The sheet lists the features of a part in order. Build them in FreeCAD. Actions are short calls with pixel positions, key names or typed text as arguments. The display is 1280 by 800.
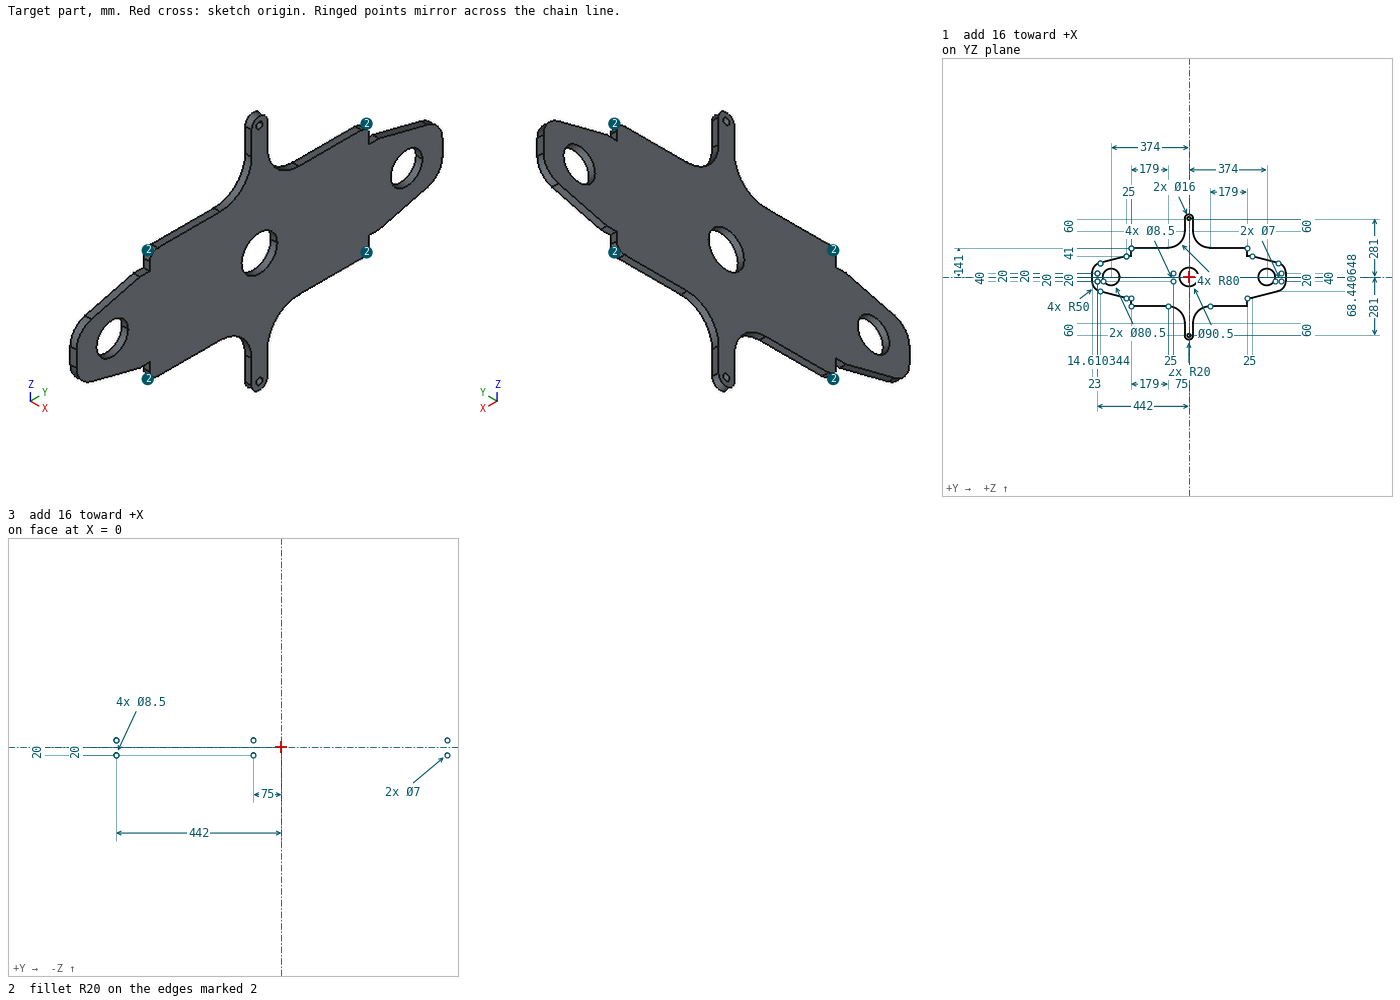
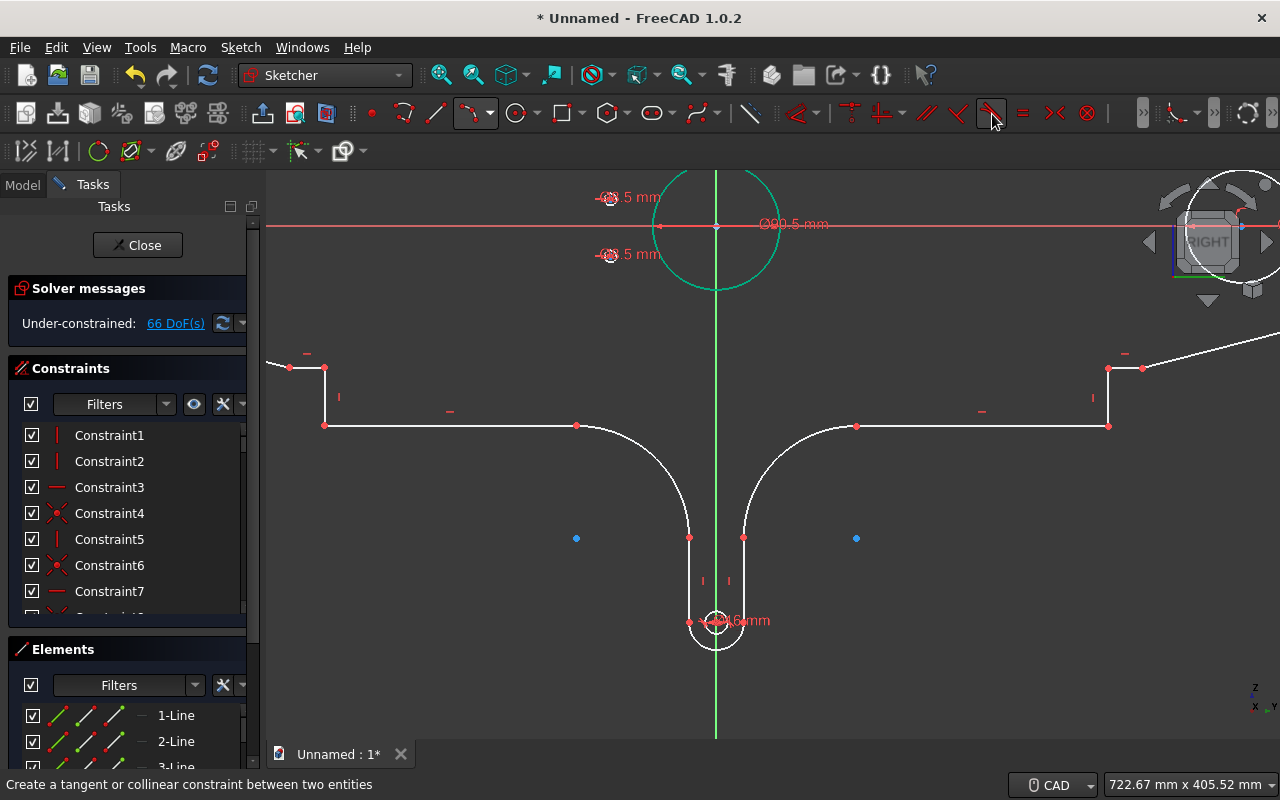
scroll(695, 641, down, 4)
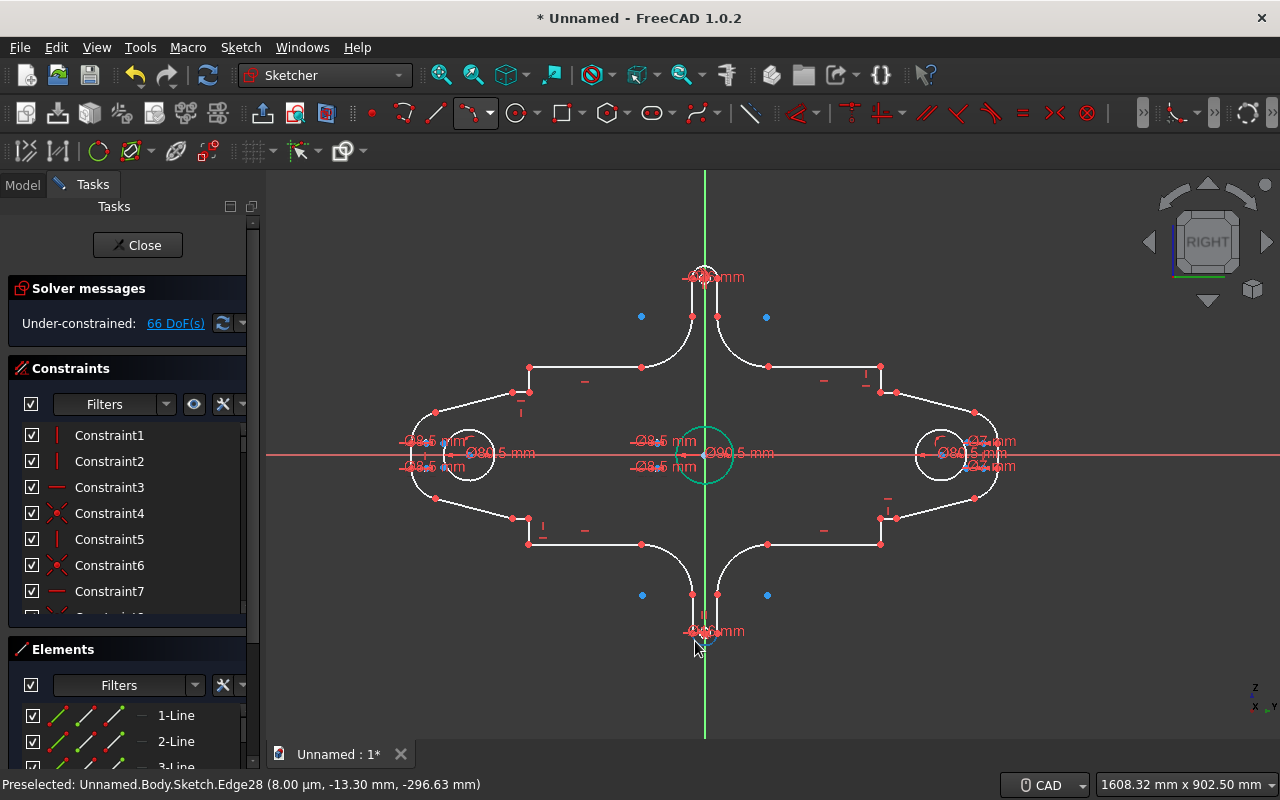
click(424, 418)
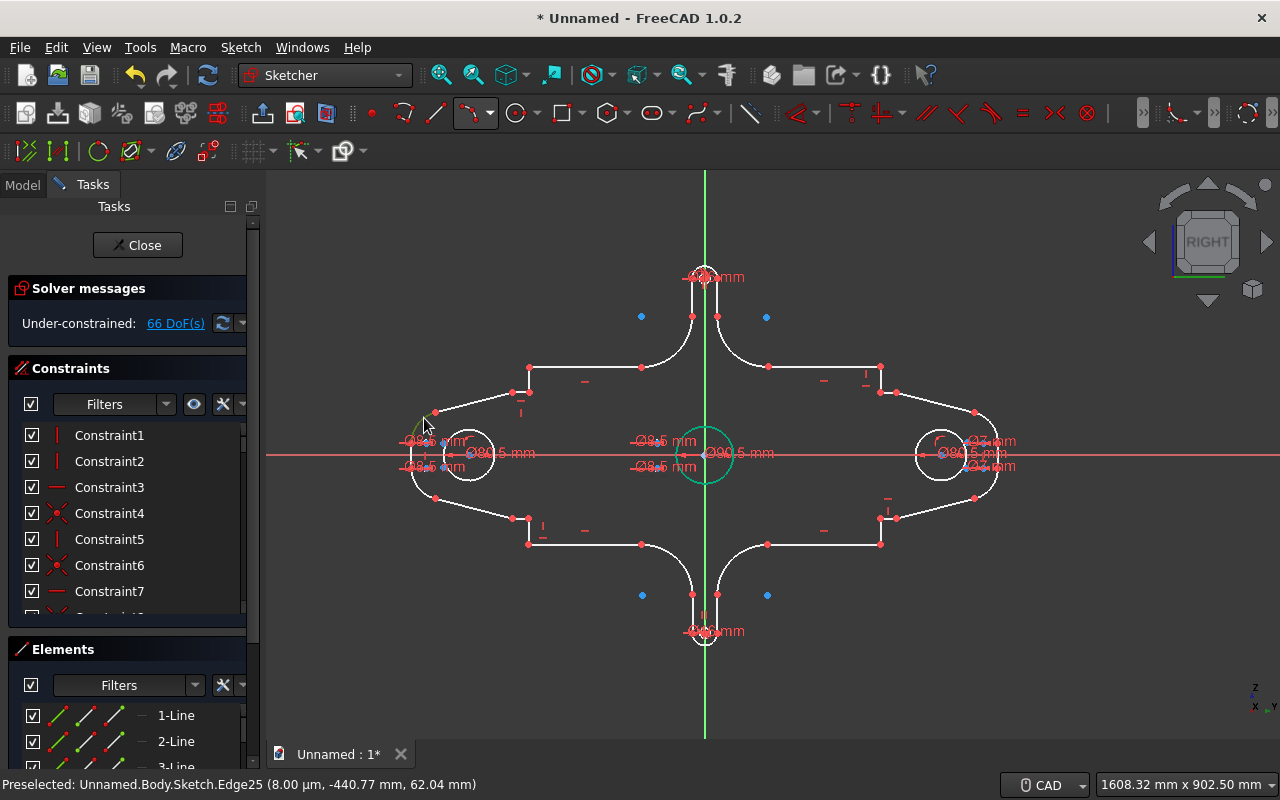
click(414, 481)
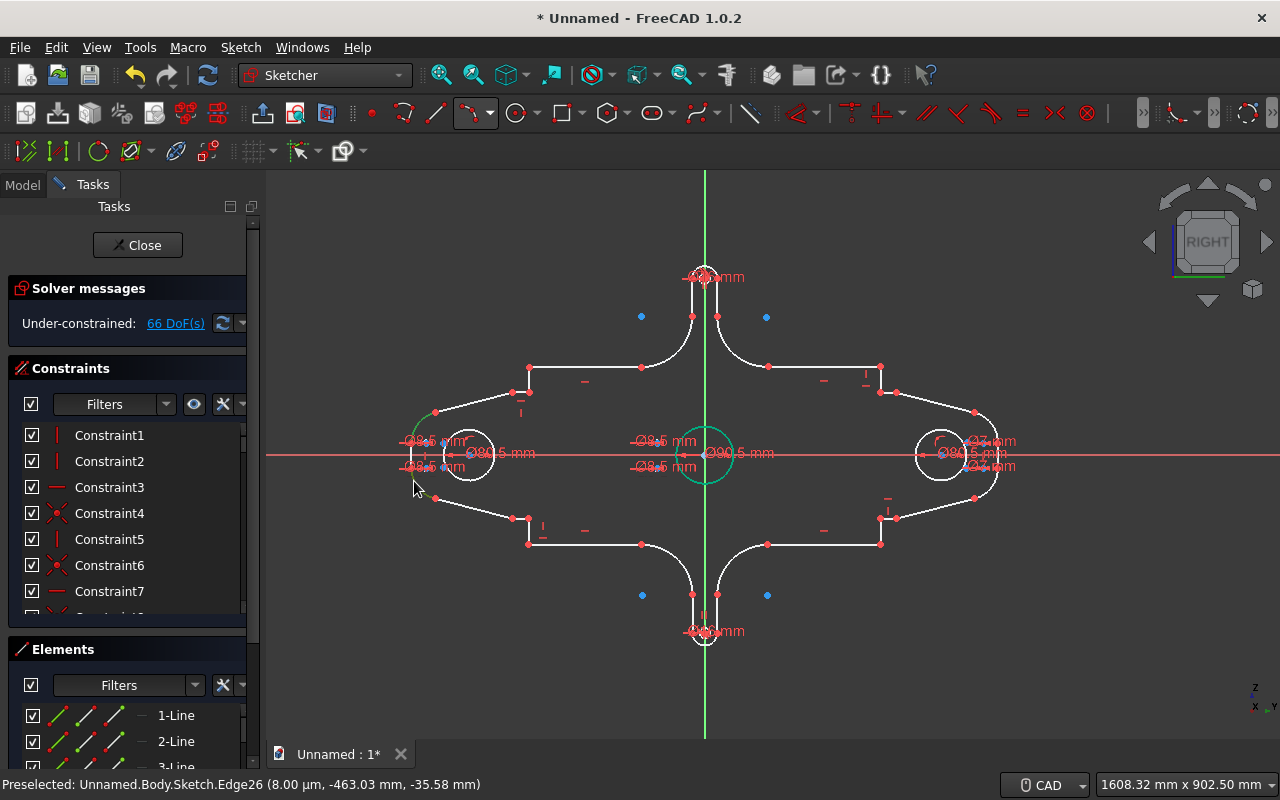
click(986, 493)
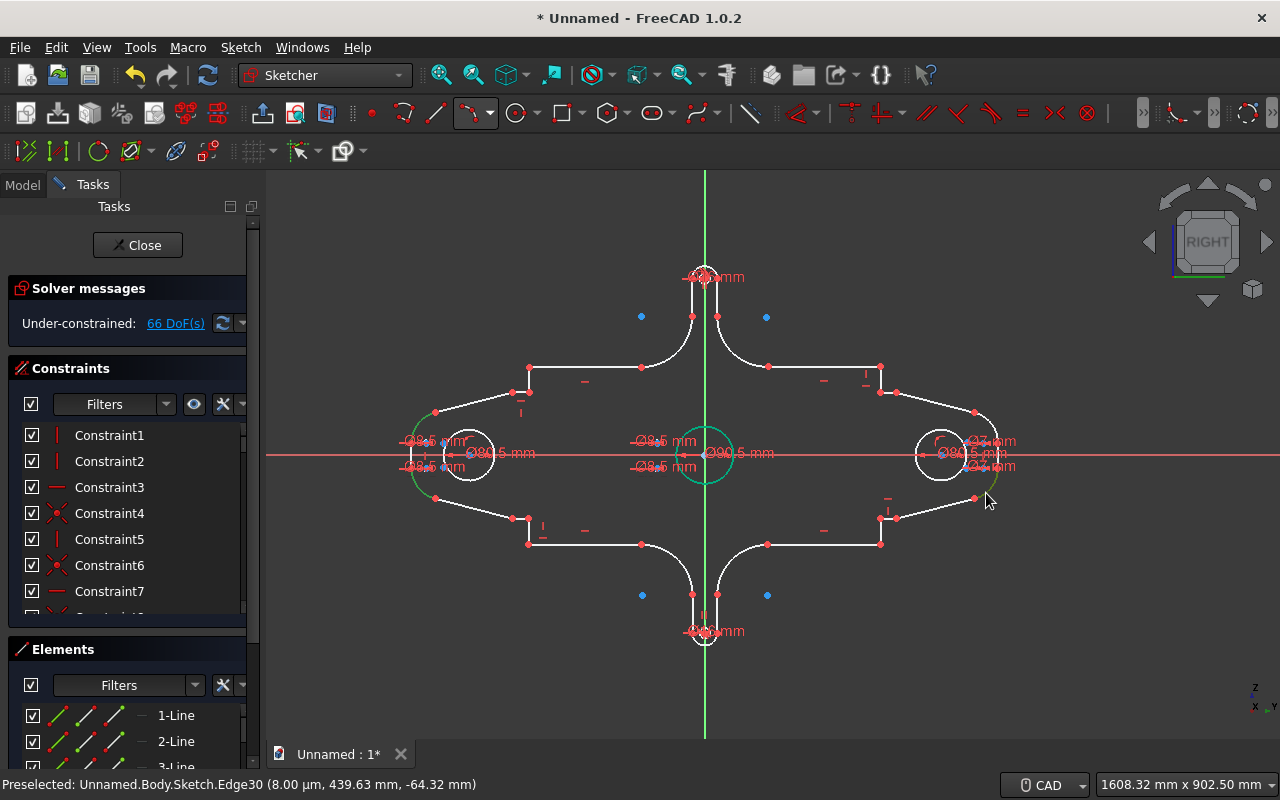
click(996, 431)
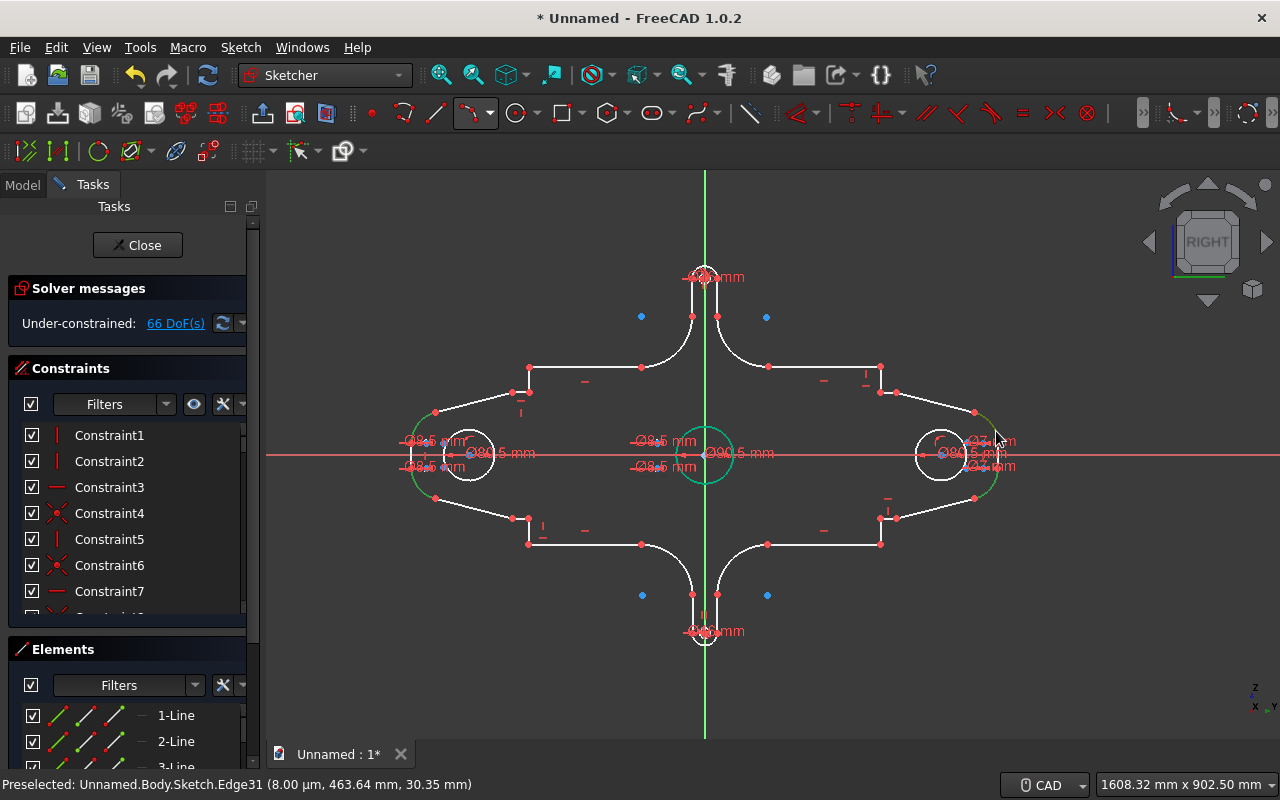
key(e)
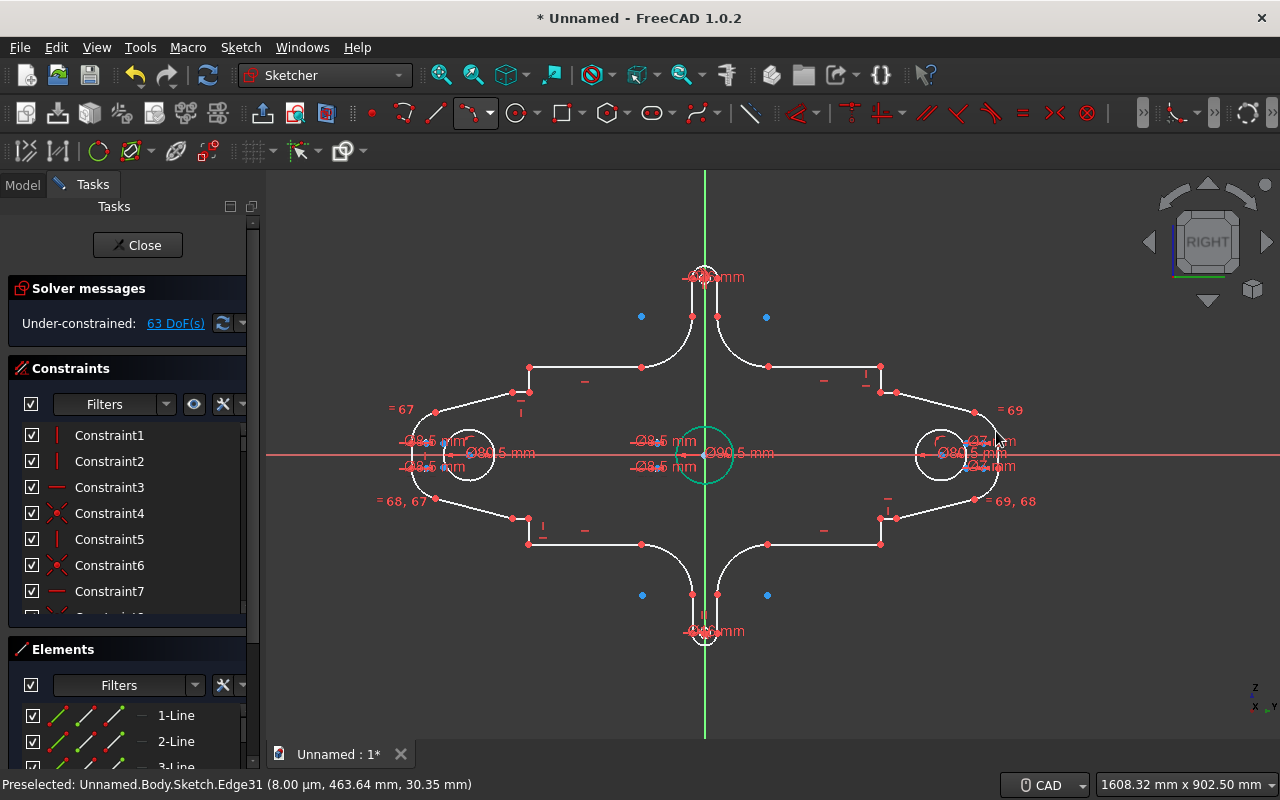
click(665, 361)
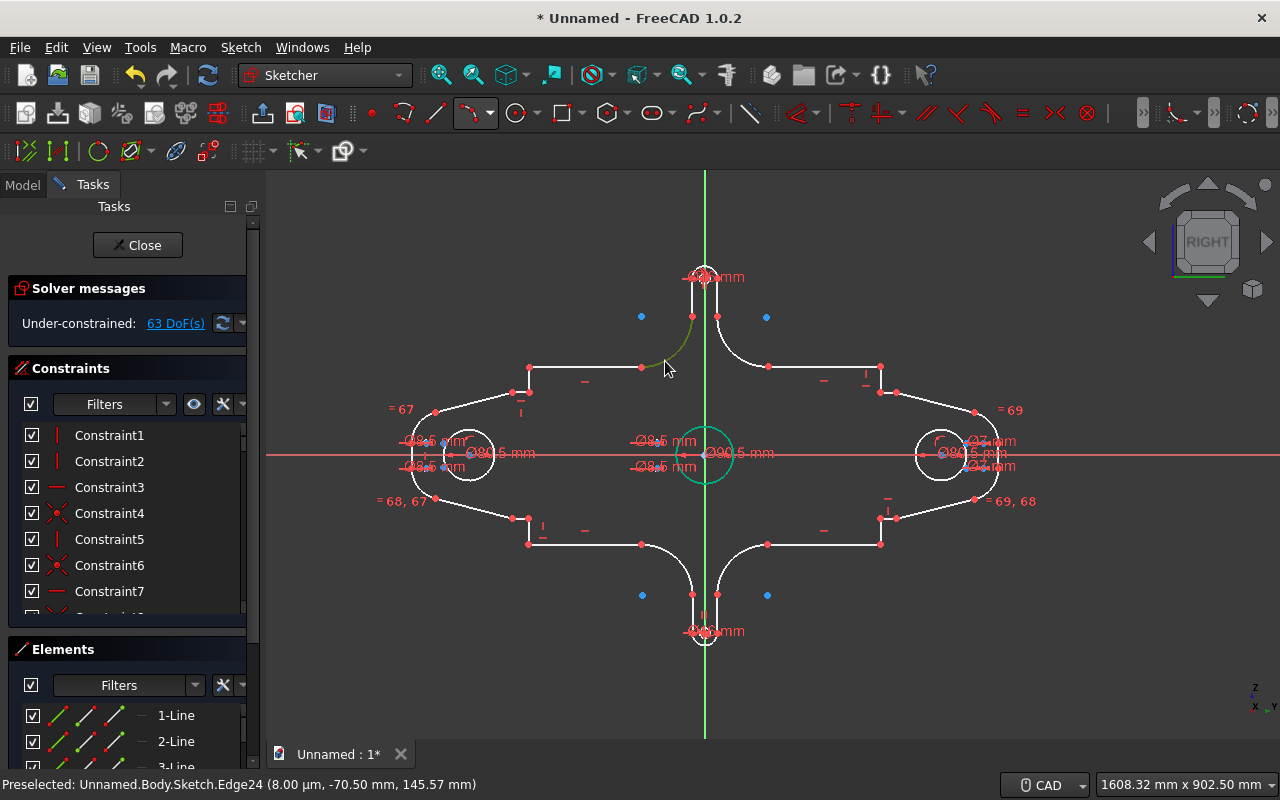
click(687, 572)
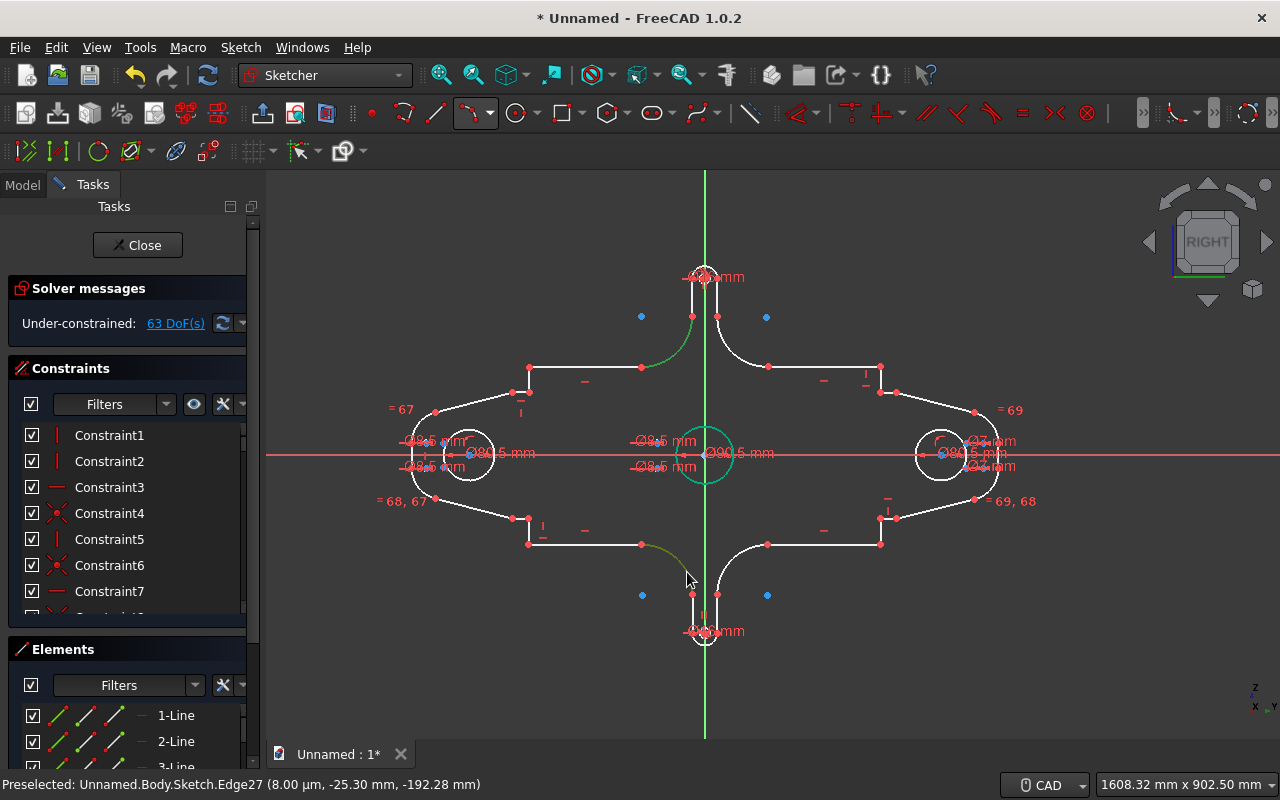
click(745, 550)